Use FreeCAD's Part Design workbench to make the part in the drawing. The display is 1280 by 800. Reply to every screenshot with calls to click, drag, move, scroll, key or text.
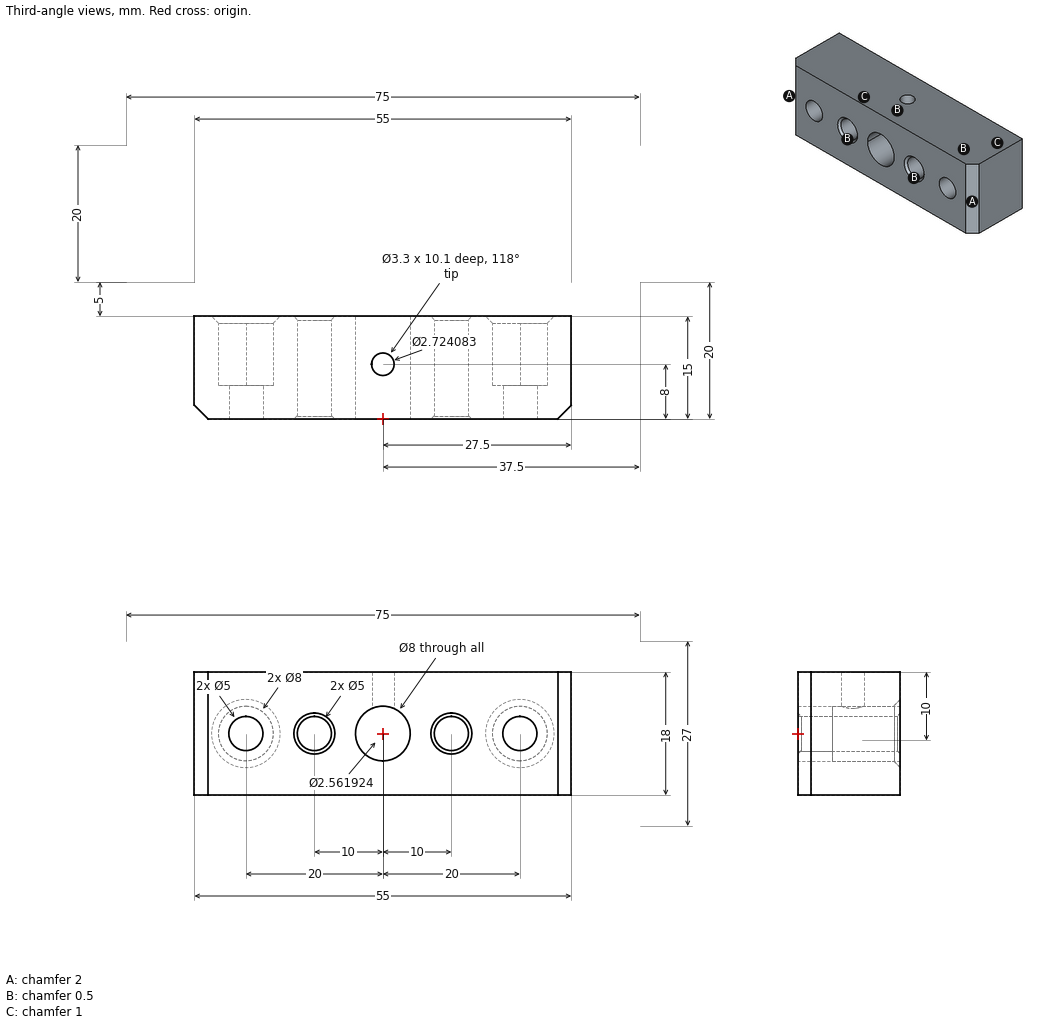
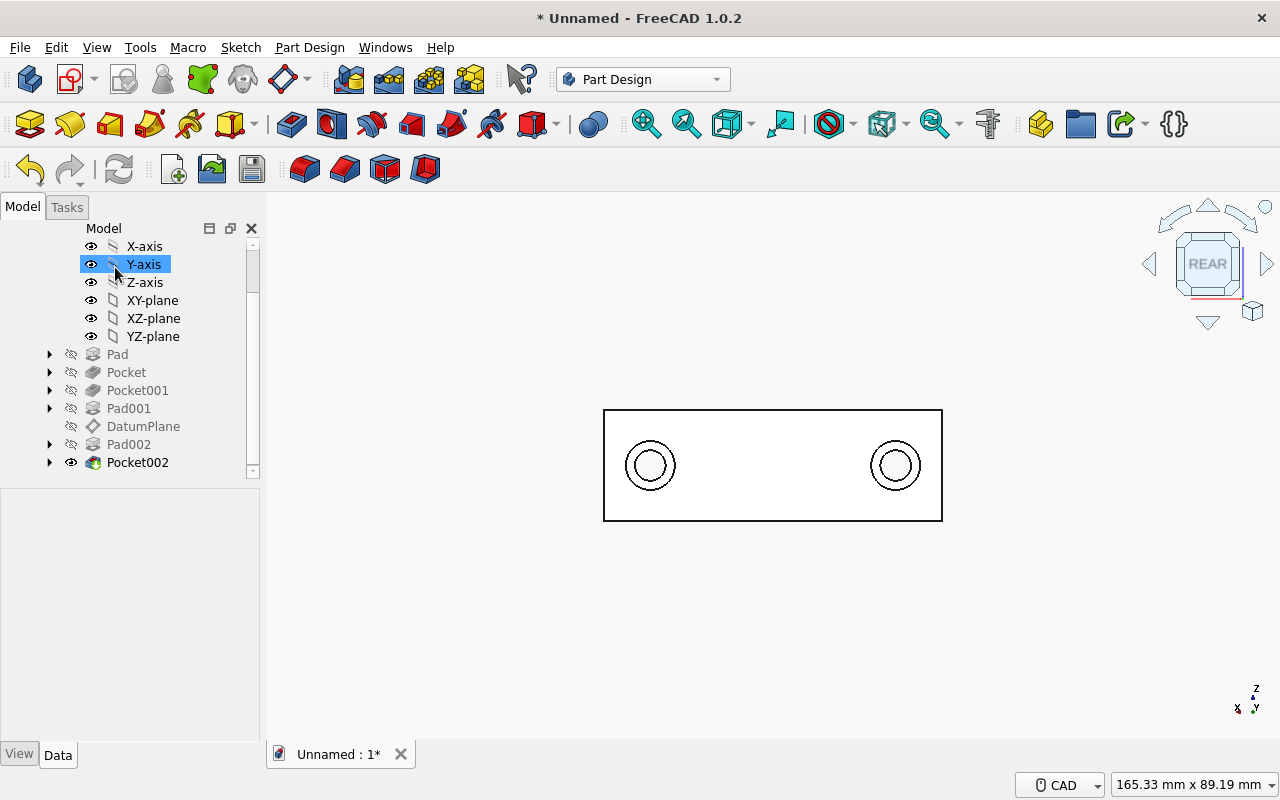
click(648, 124)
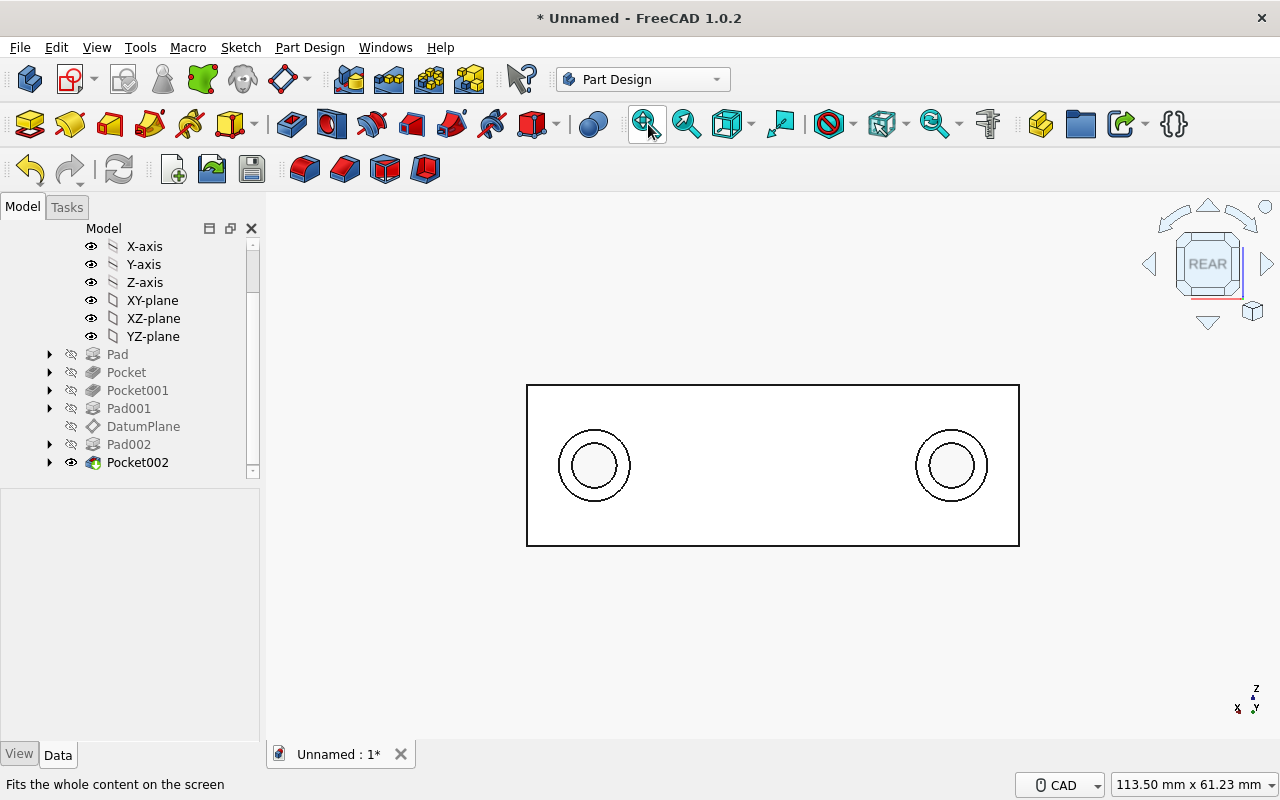
click(773, 465)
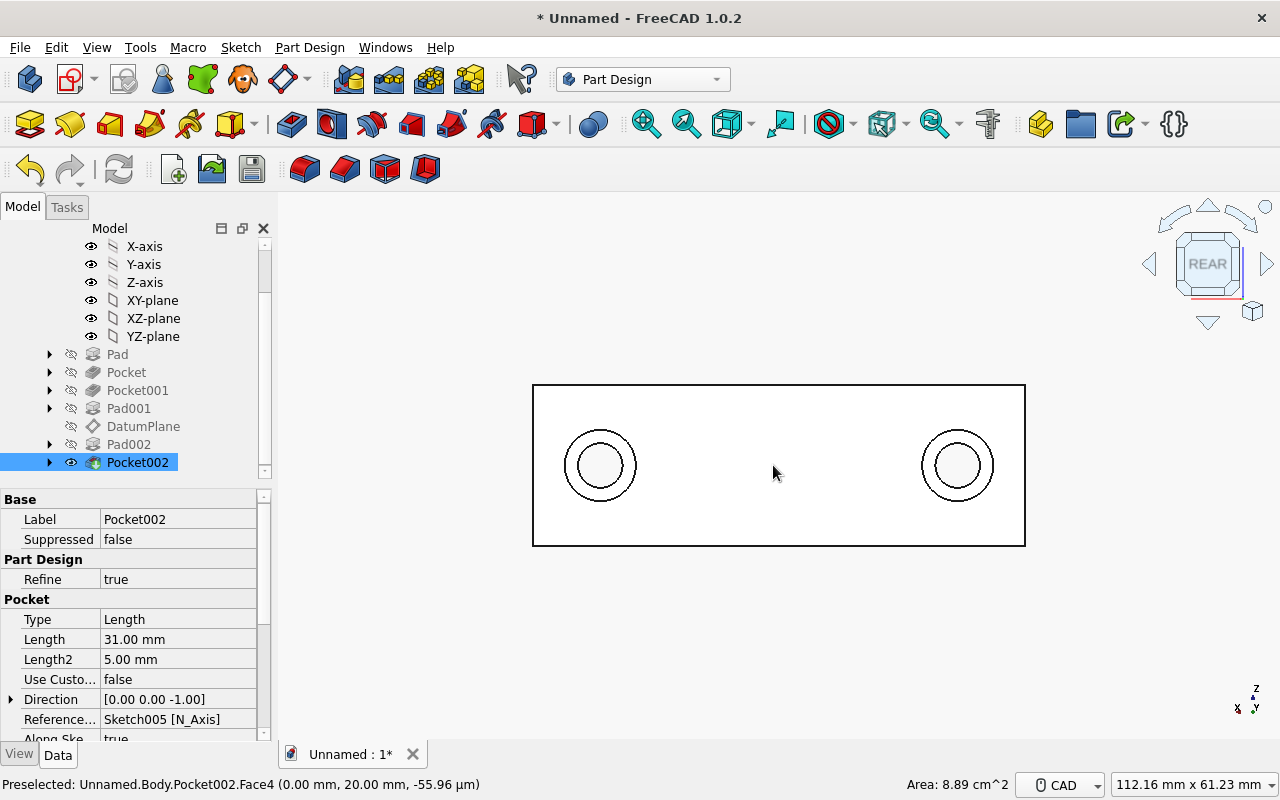
click(70, 80)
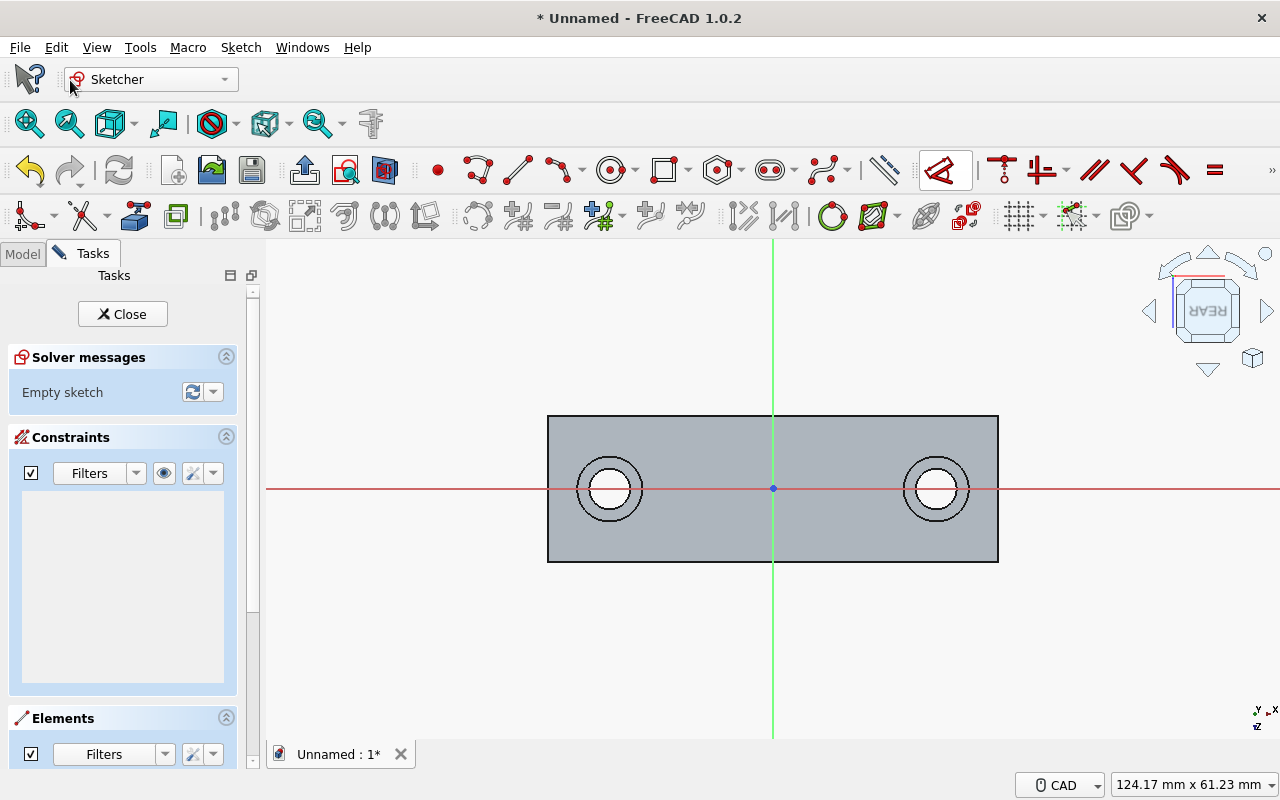
scroll(777, 489, up, 14)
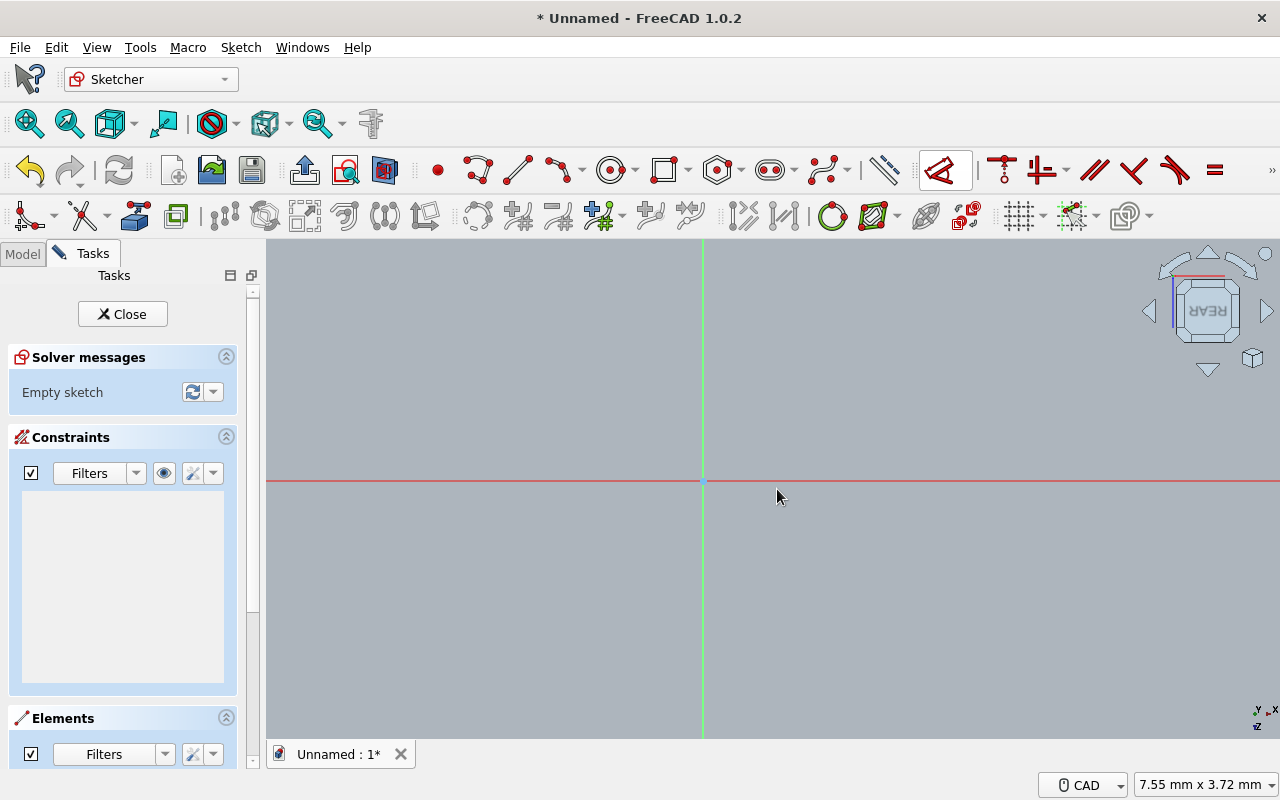
click(612, 170)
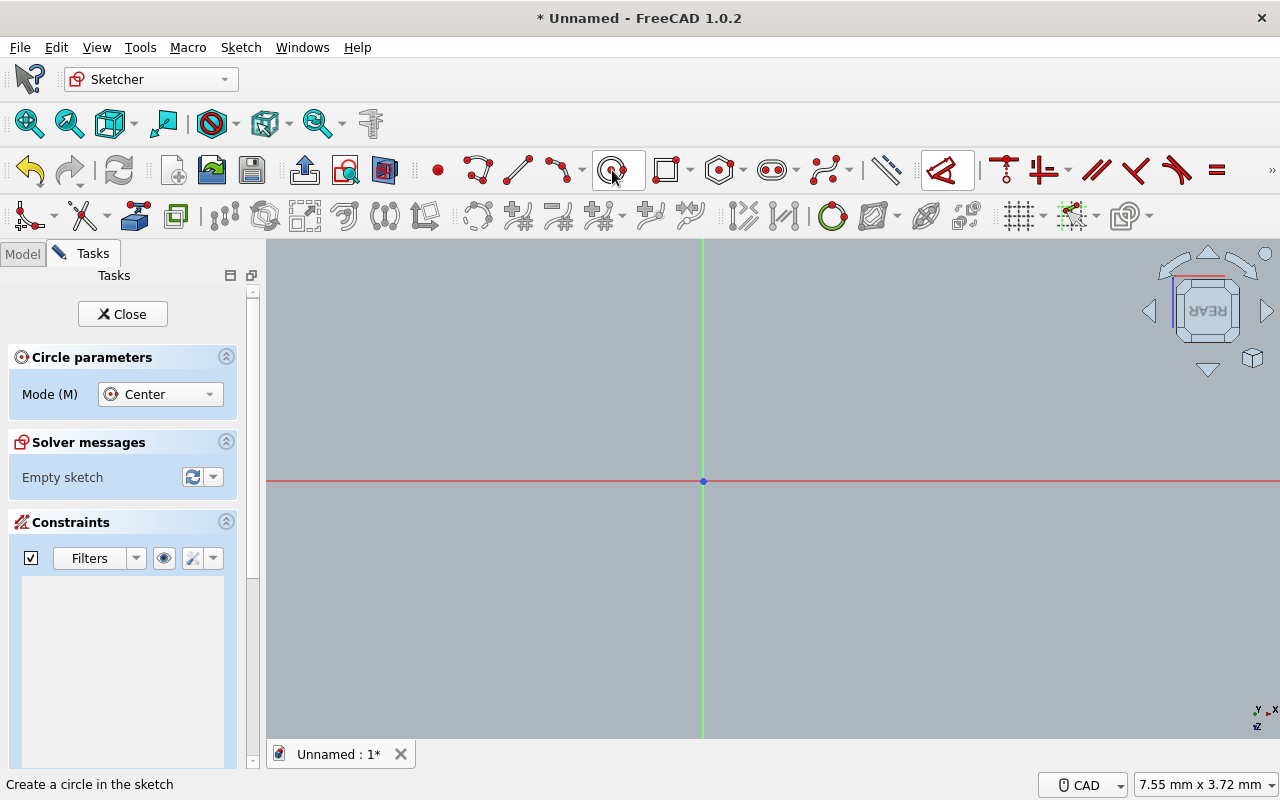
click(703, 481)
move(825, 360)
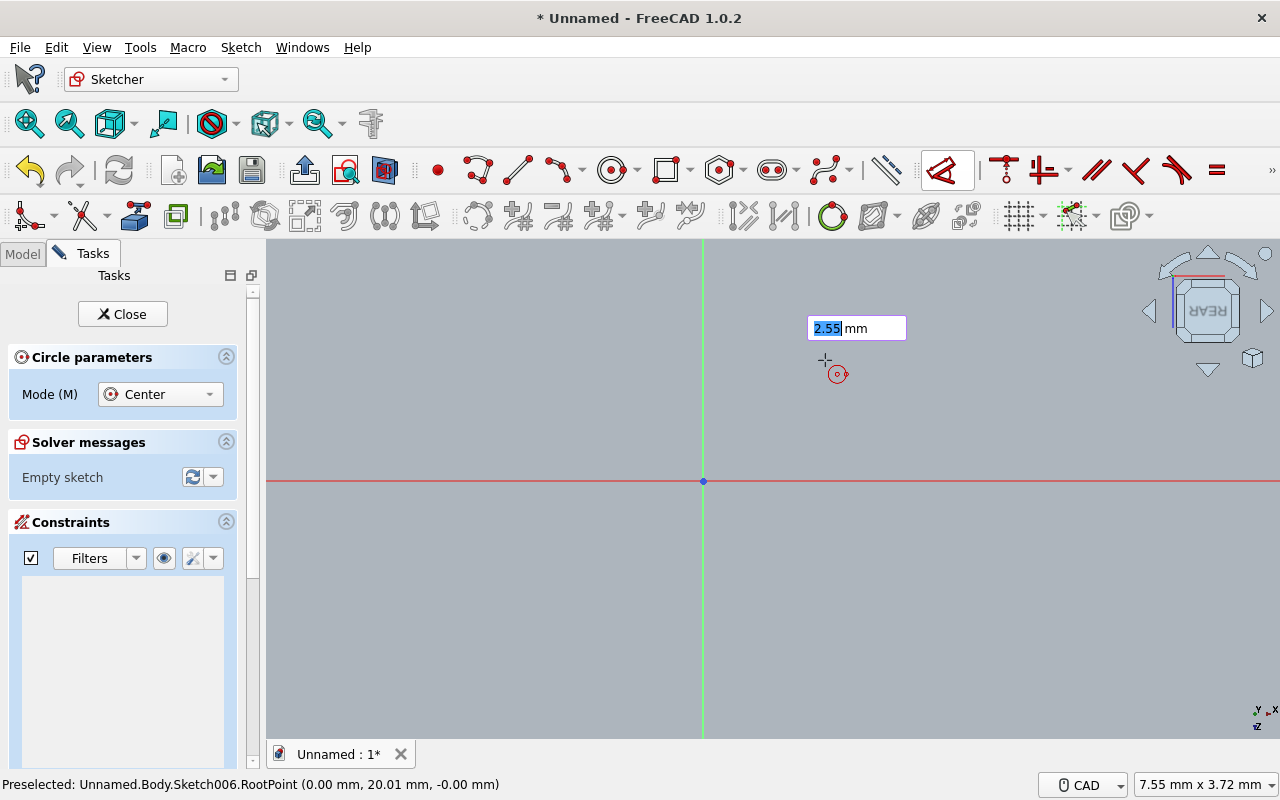
text(2.561924)
key(Return)
key(Escape)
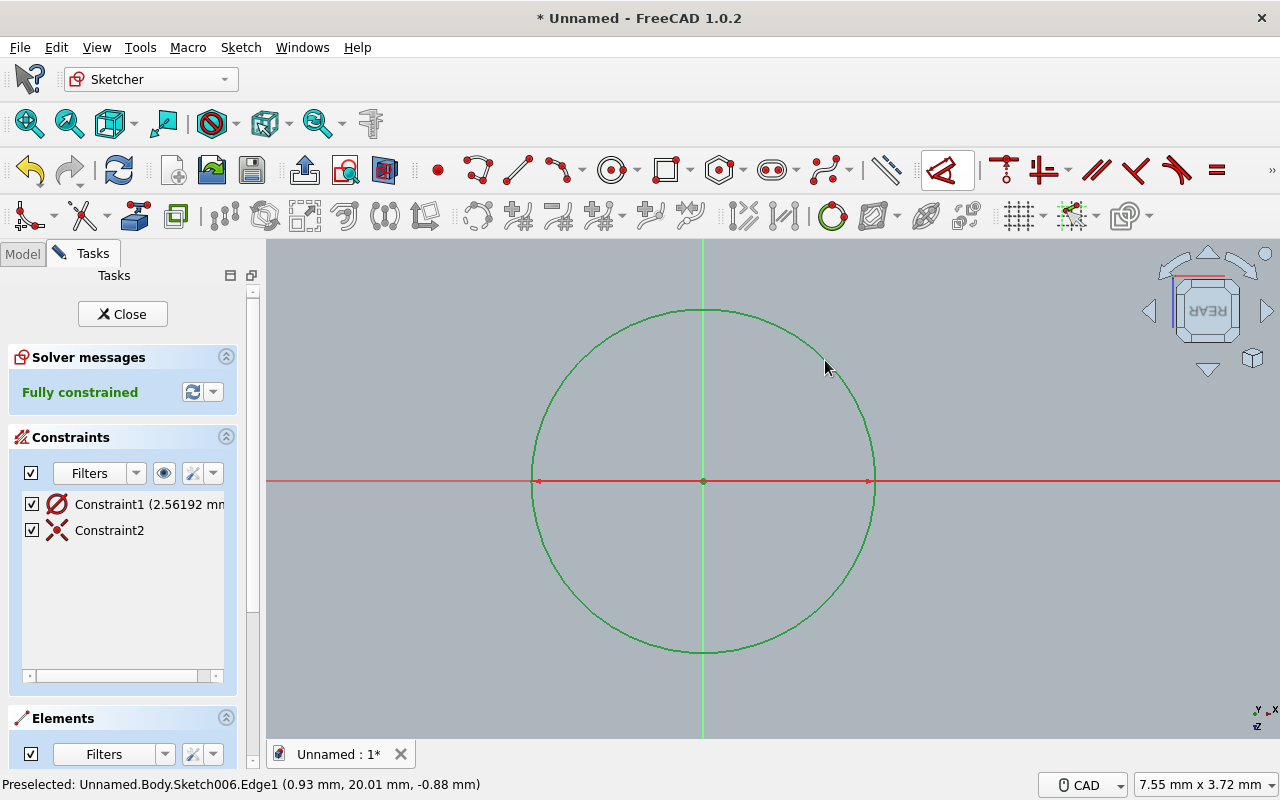
click(123, 314)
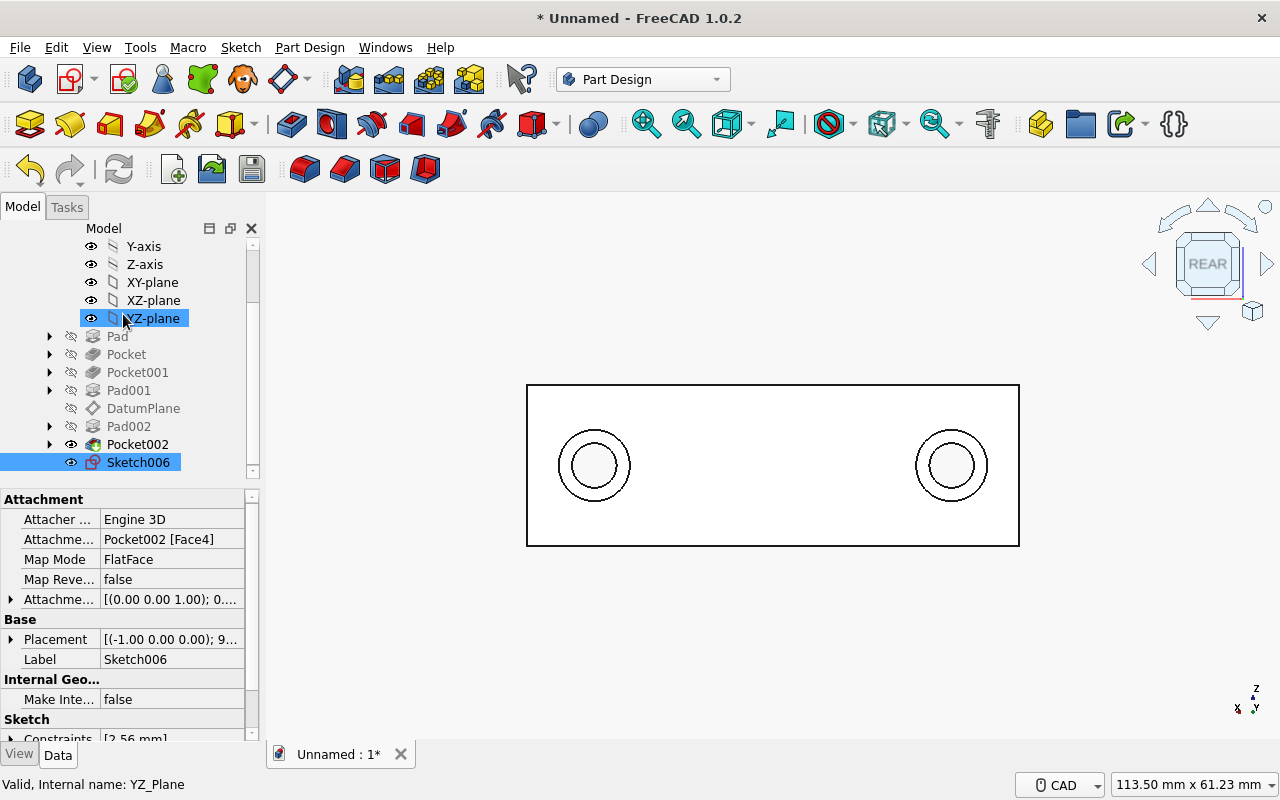
click(292, 124)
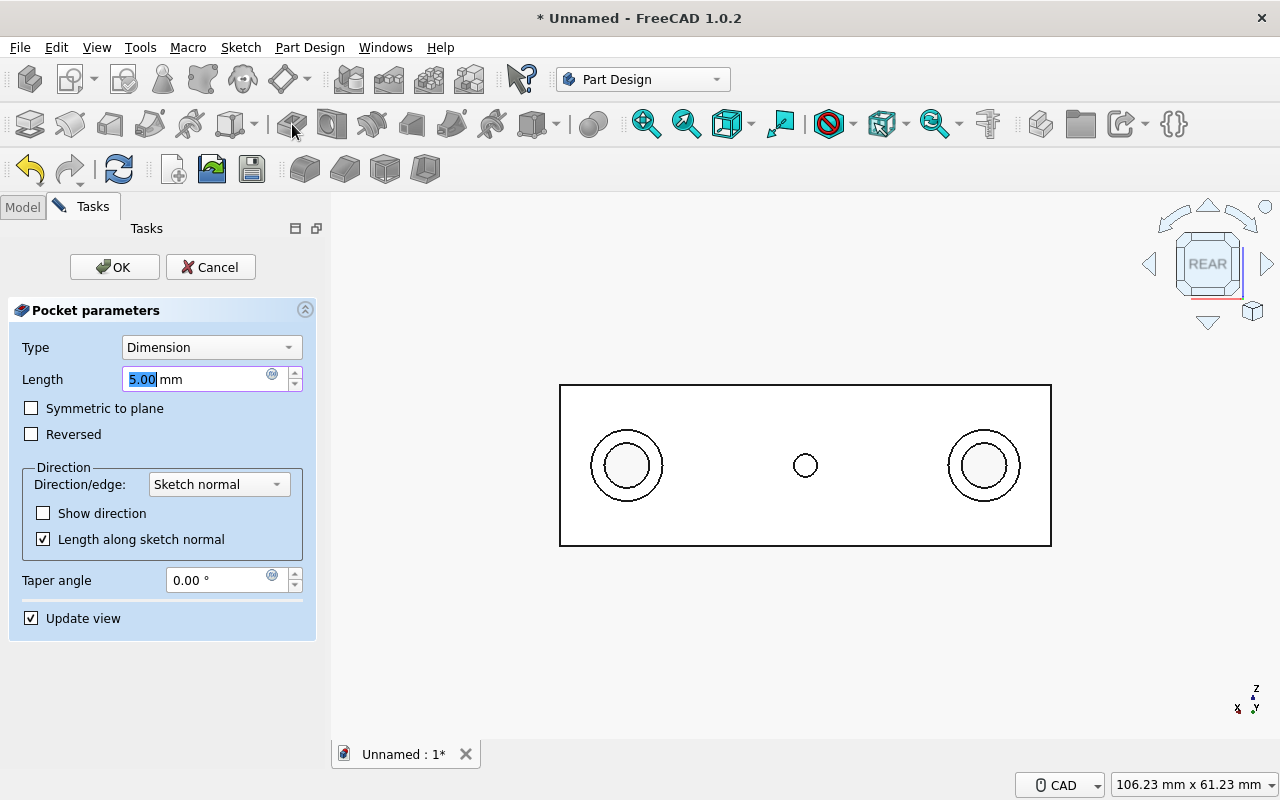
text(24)
key(Tab)